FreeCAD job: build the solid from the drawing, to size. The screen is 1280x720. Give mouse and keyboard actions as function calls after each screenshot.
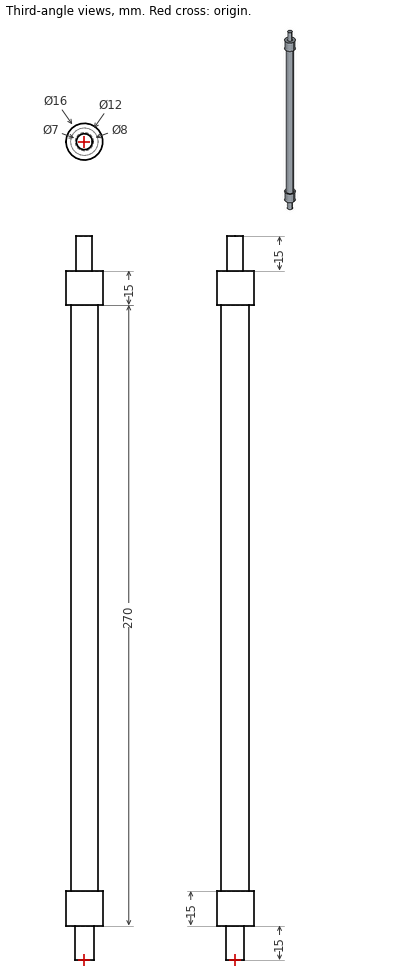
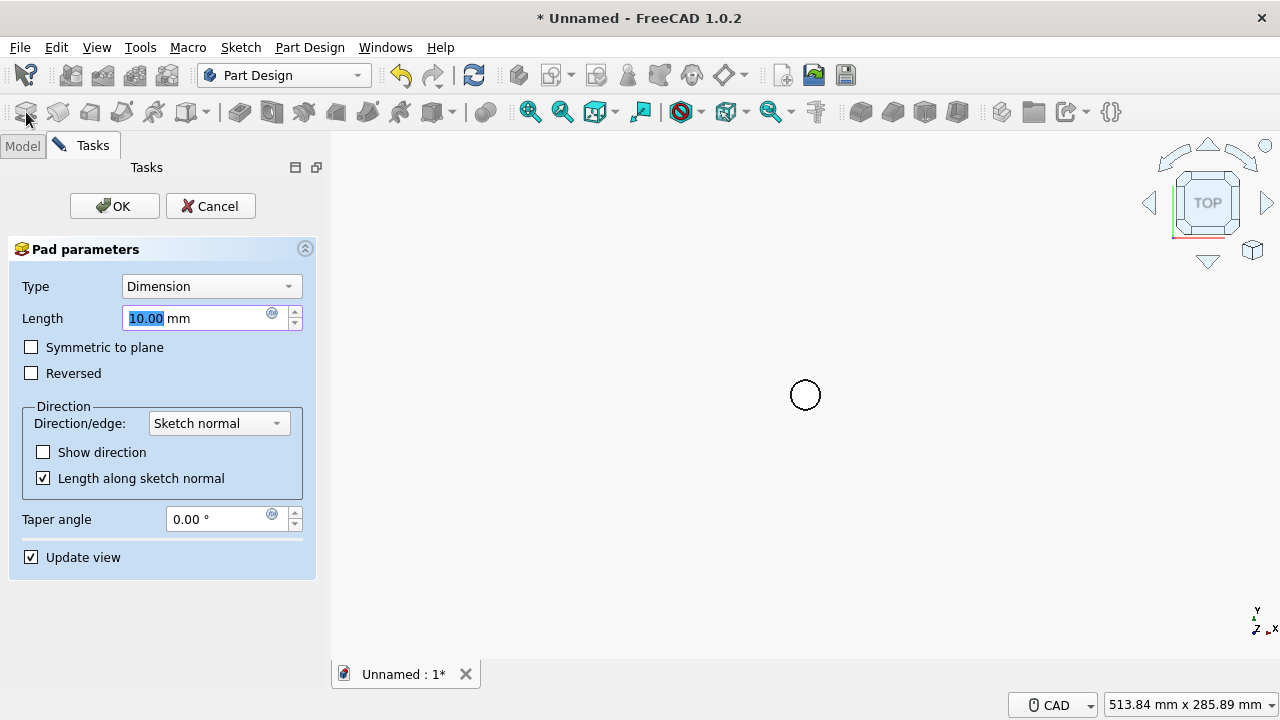
text(15)
key(Tab)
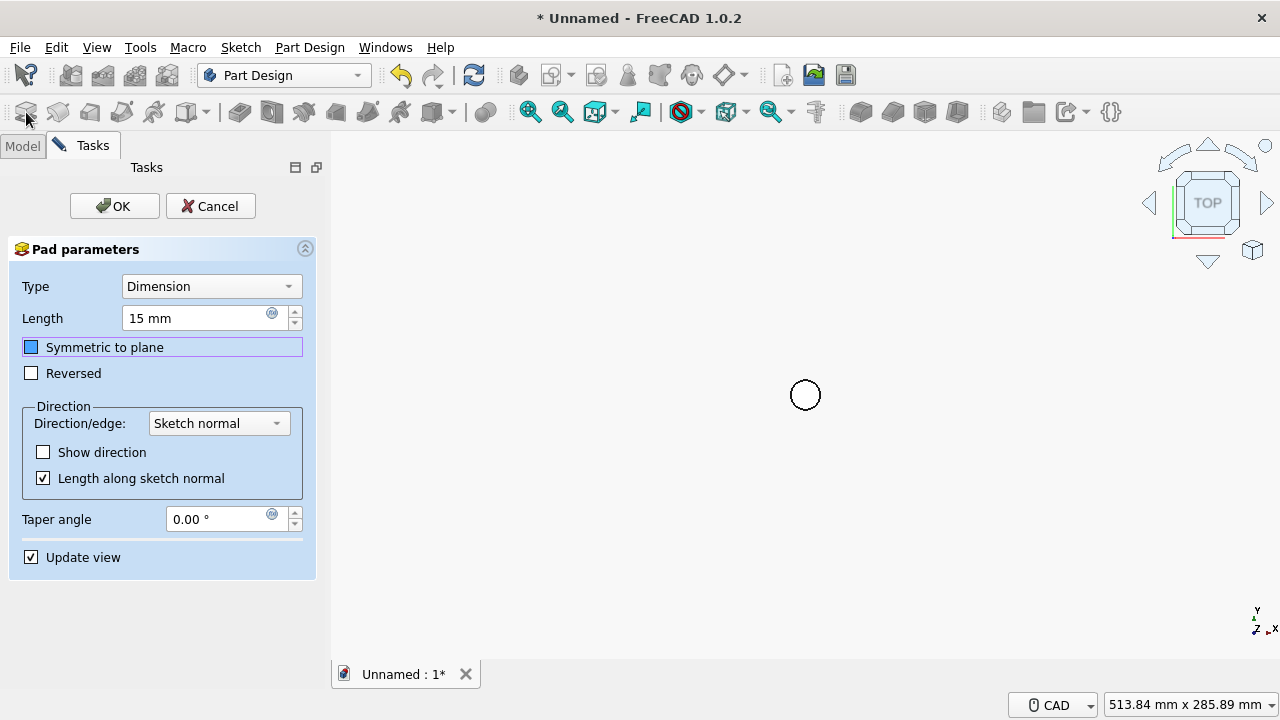
click(115, 206)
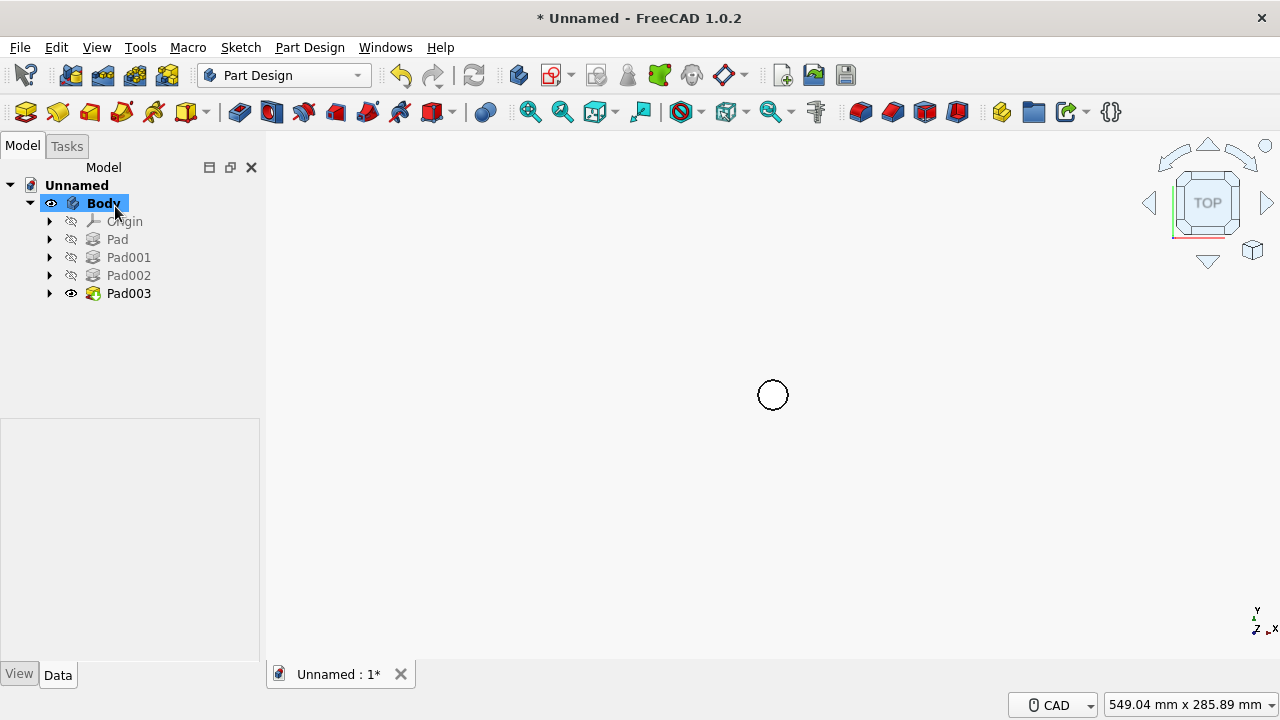
click(532, 112)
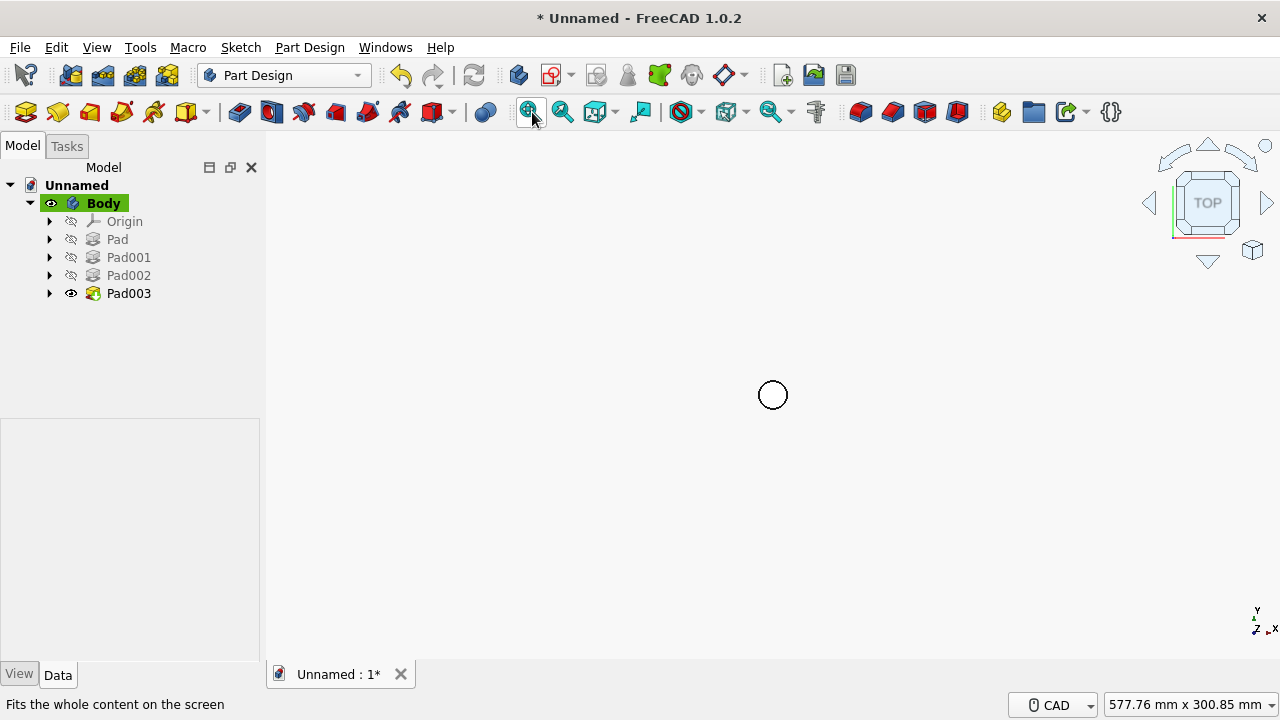
click(773, 394)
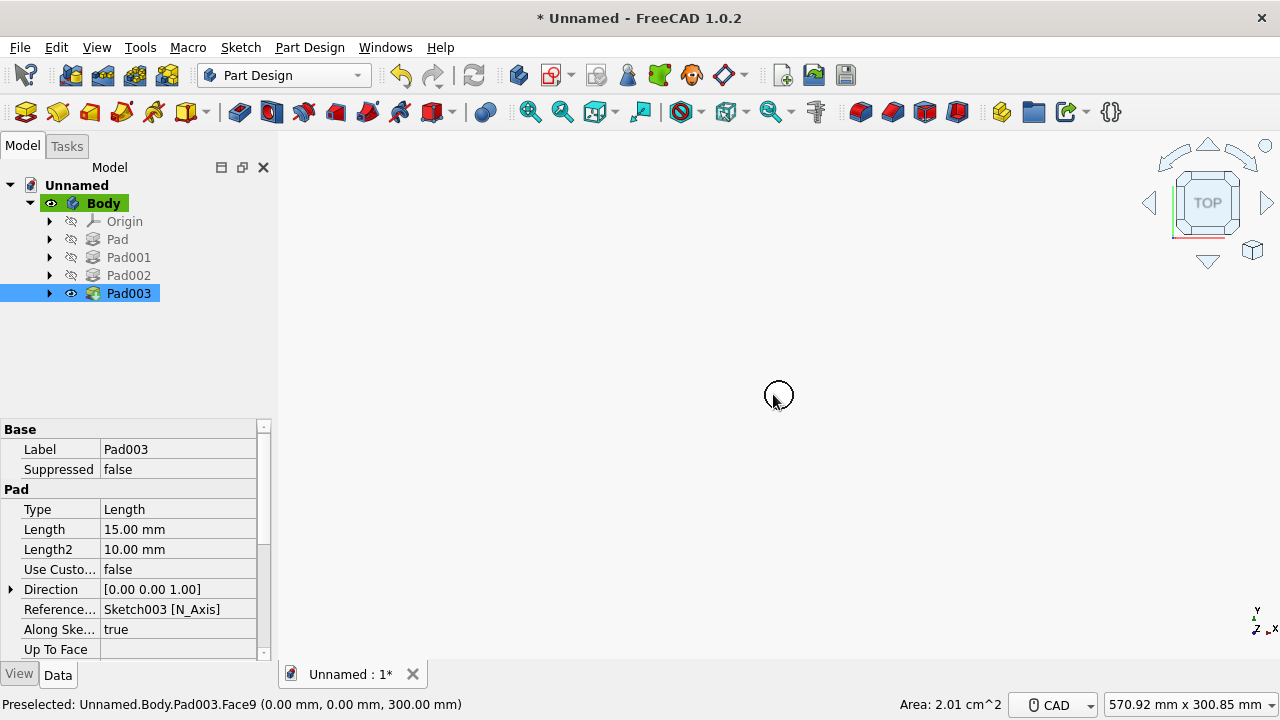
click(552, 76)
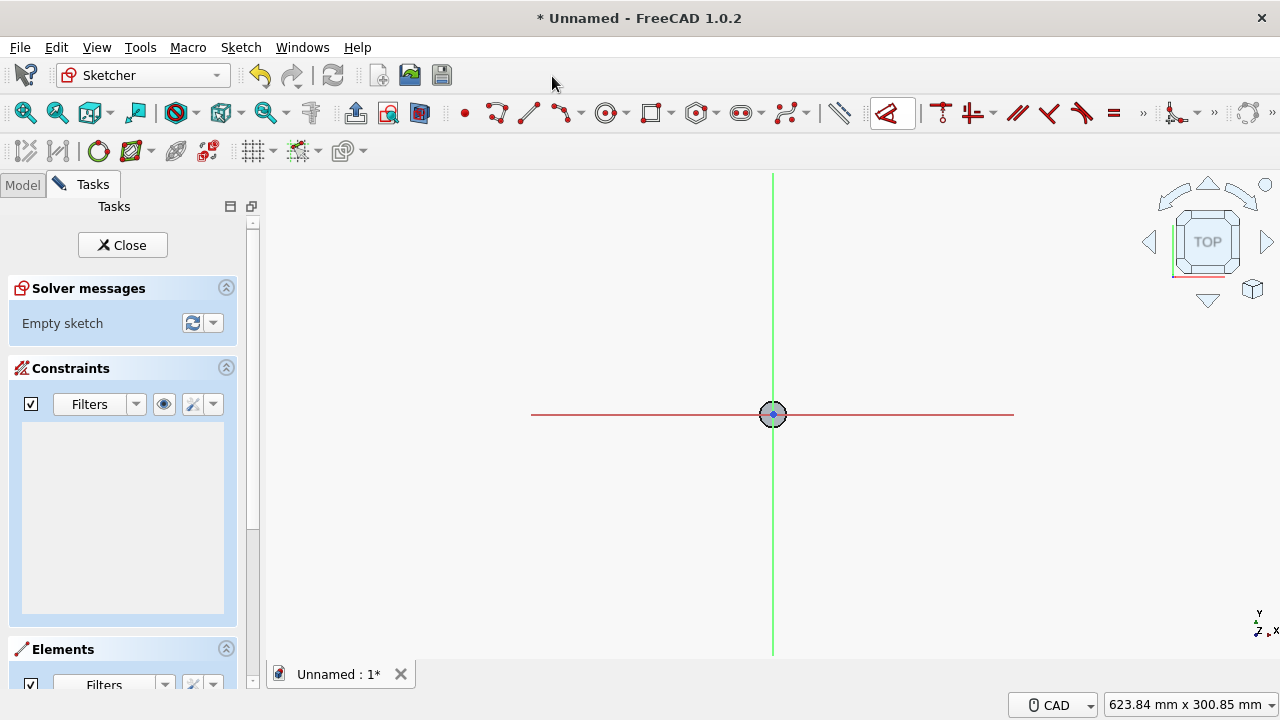
scroll(777, 414, up, 15)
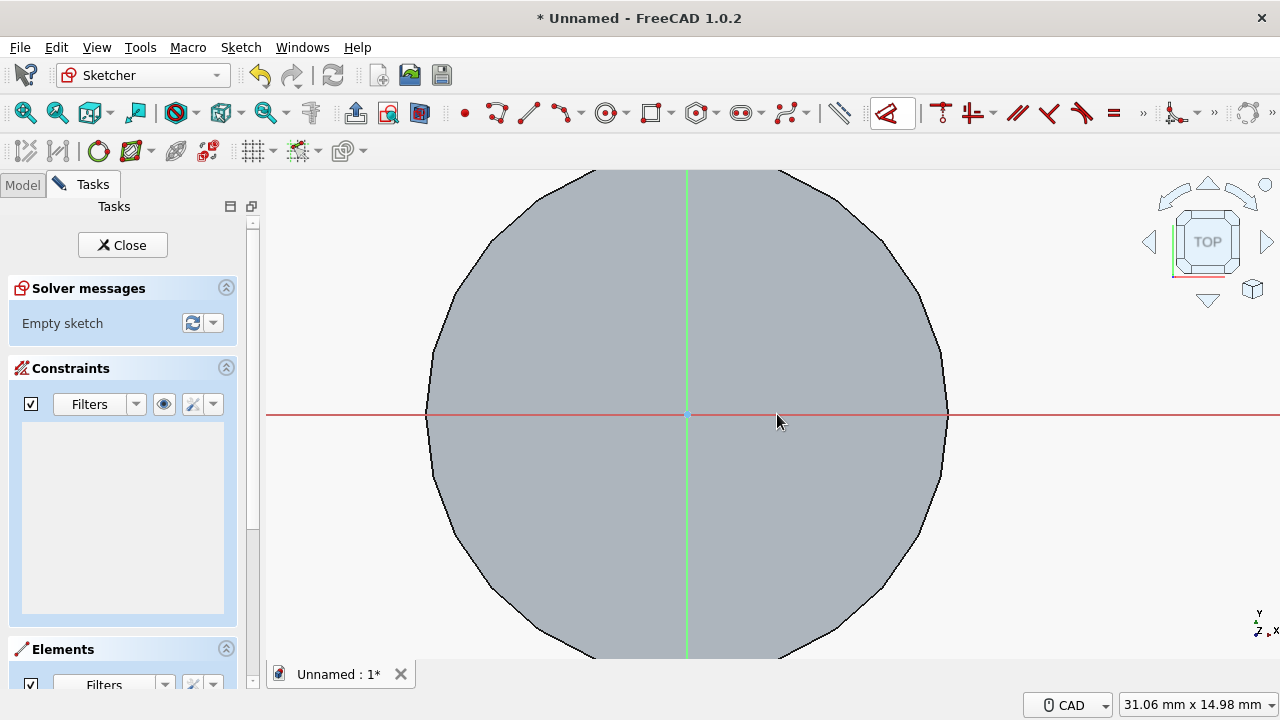
click(606, 114)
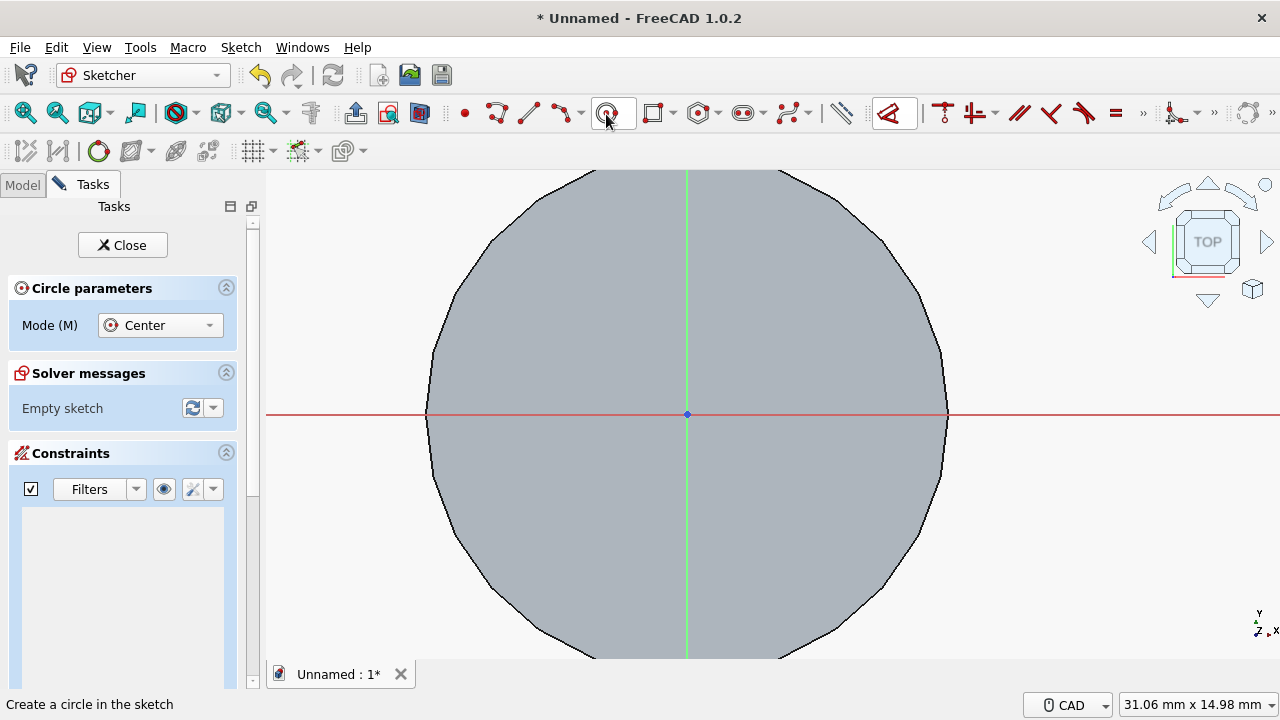
click(687, 414)
click(768, 334)
key(Escape)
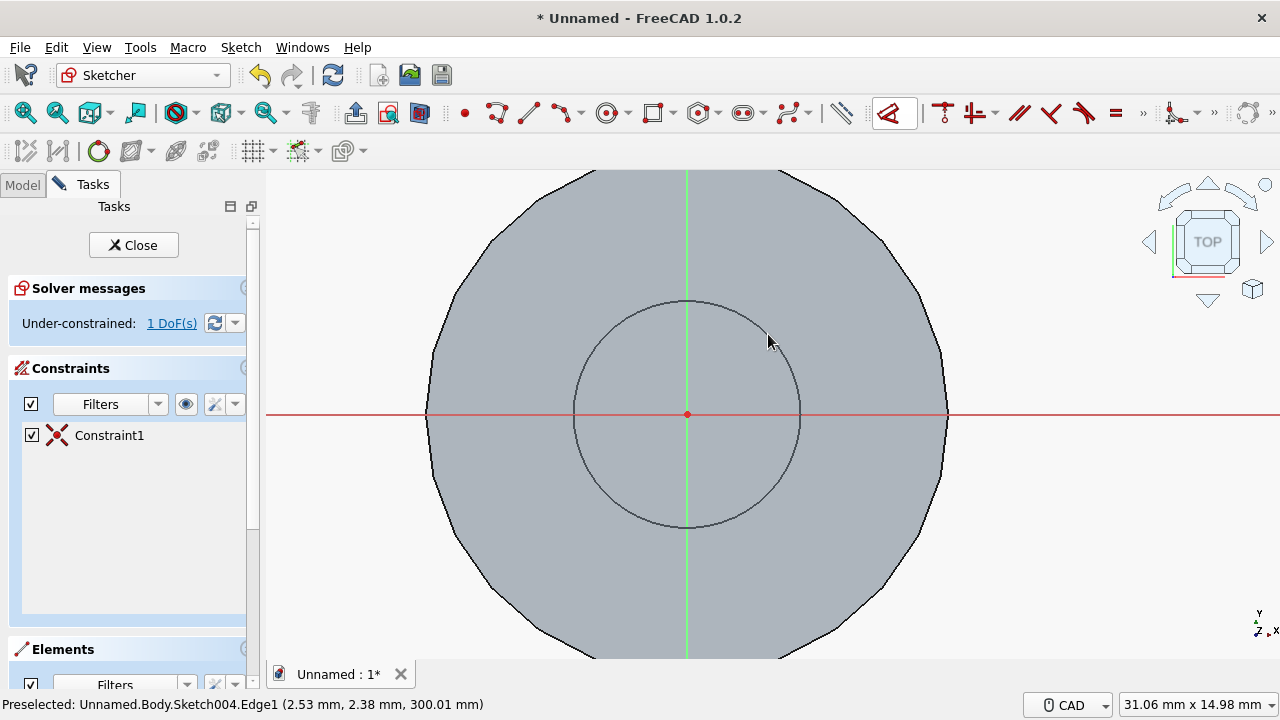
click(767, 334)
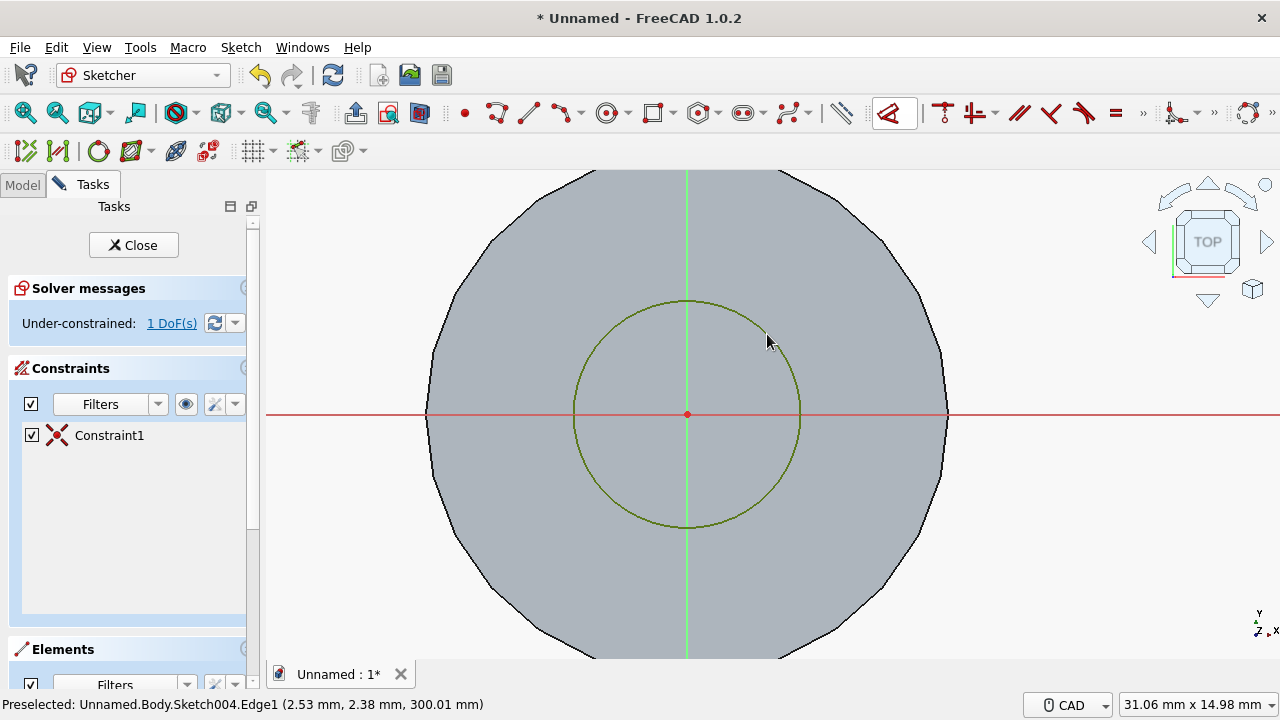
click(912, 114)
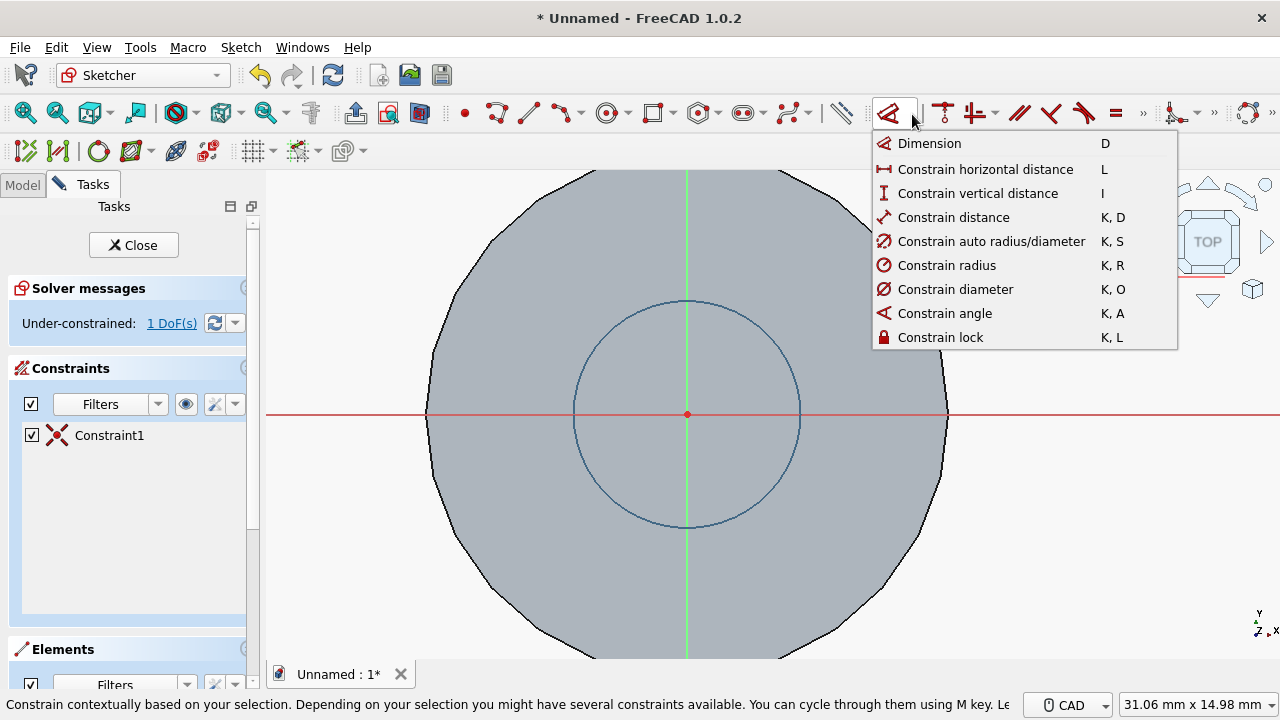
click(1025, 289)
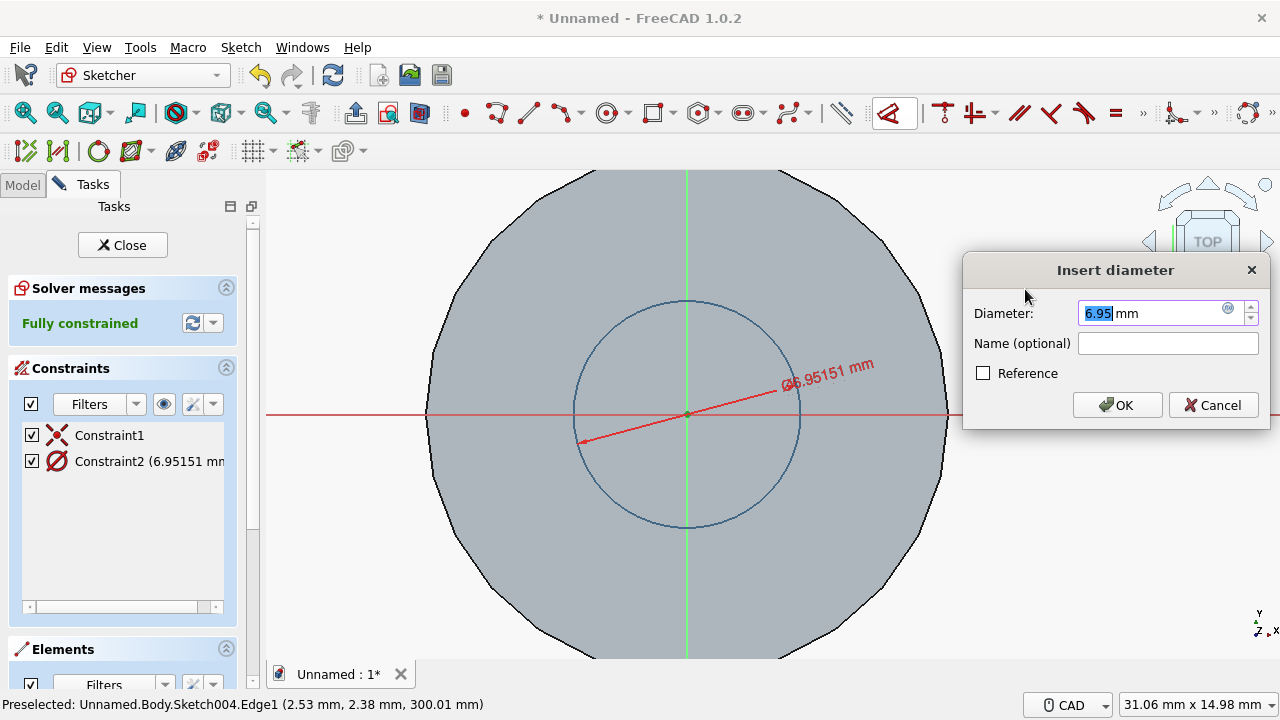
text(7)
key(Return)